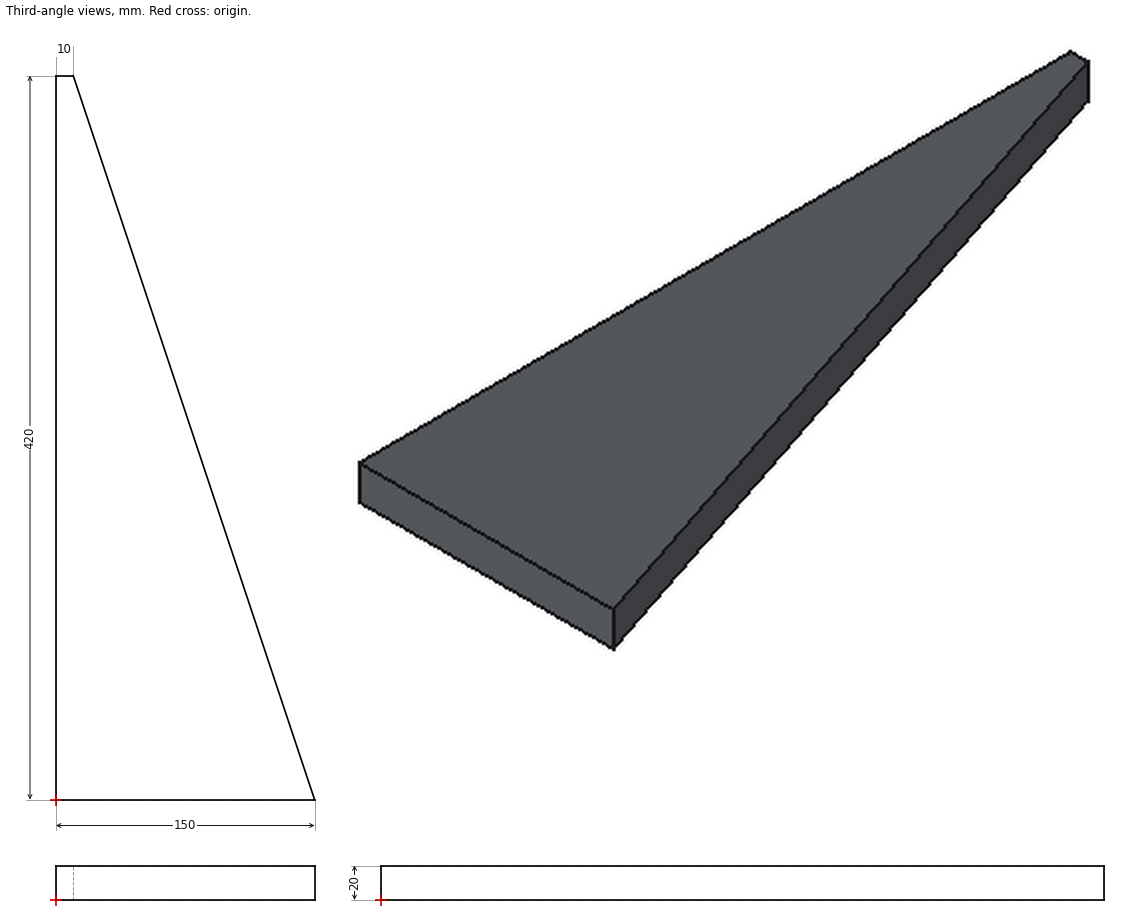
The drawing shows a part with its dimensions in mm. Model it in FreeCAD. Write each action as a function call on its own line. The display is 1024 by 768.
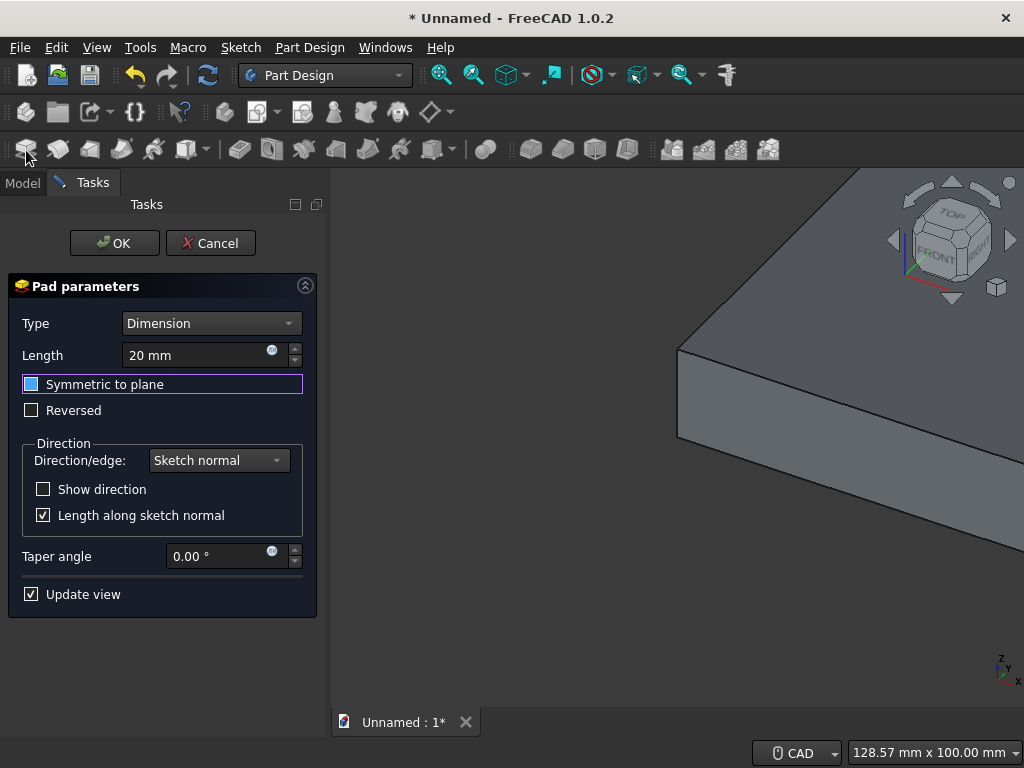
click(115, 243)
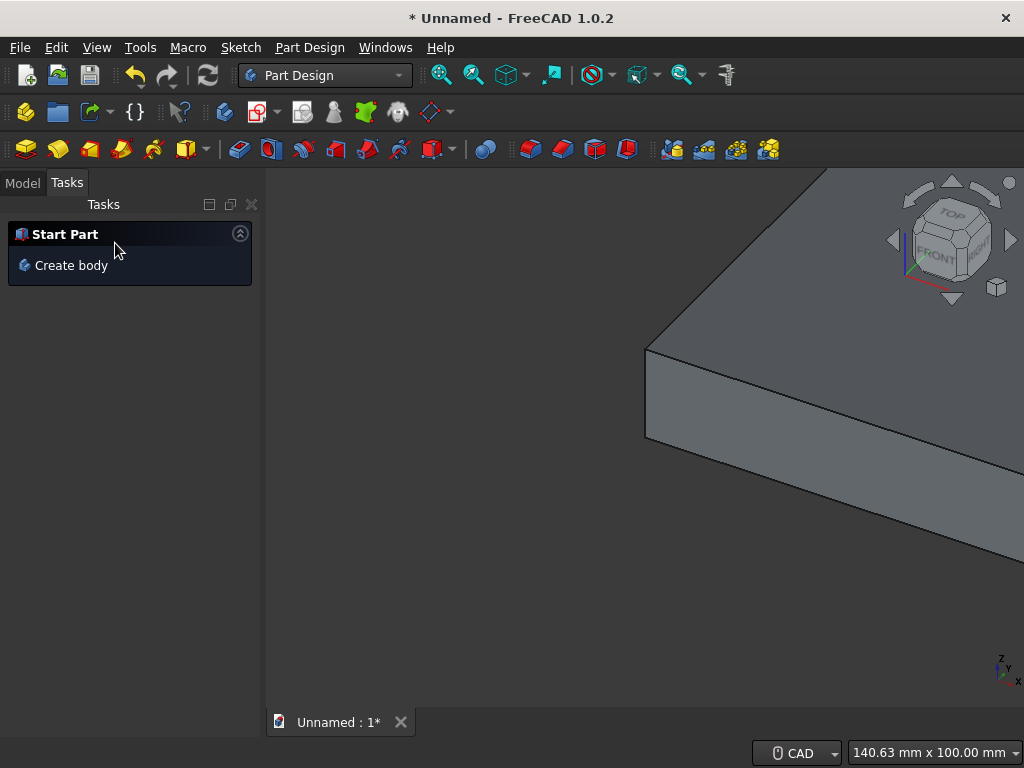
key(0)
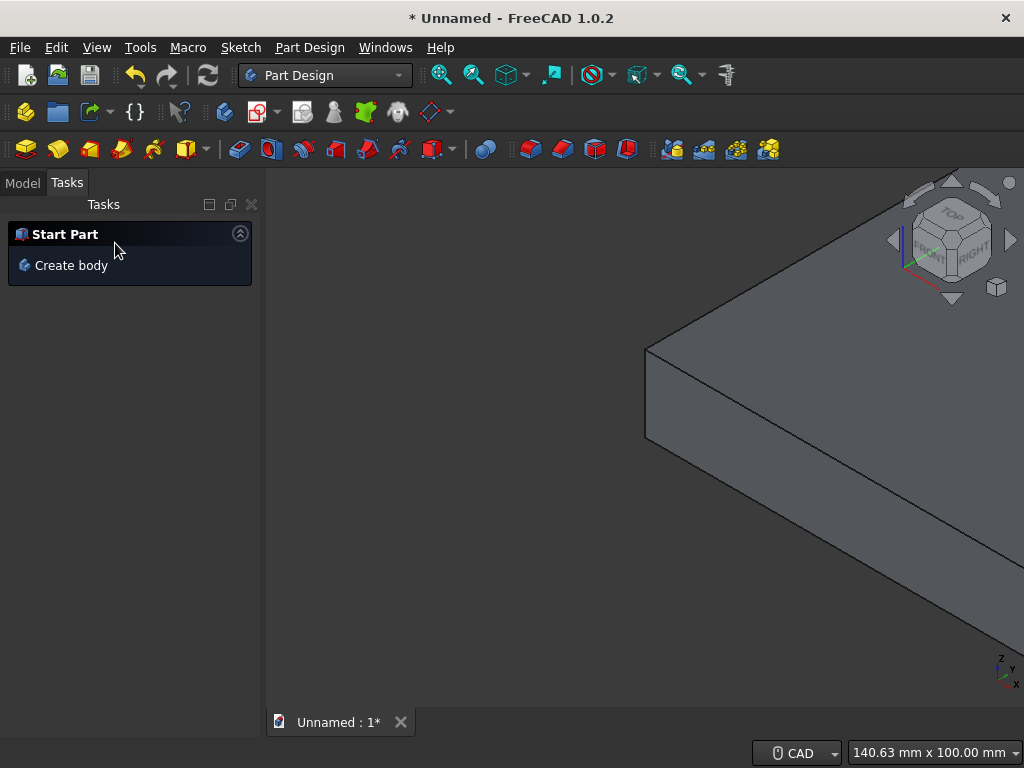
click(442, 76)